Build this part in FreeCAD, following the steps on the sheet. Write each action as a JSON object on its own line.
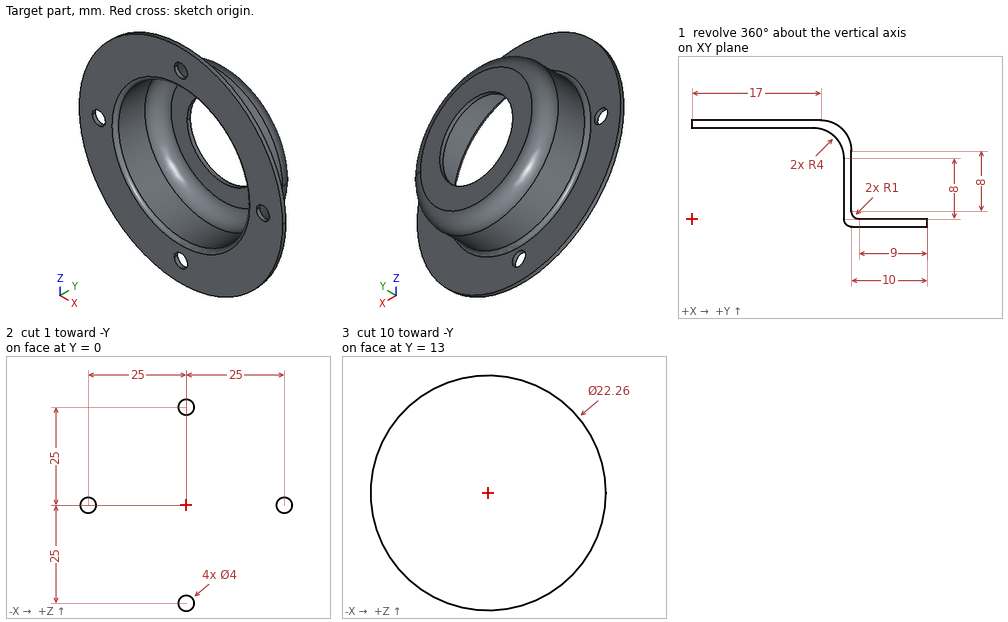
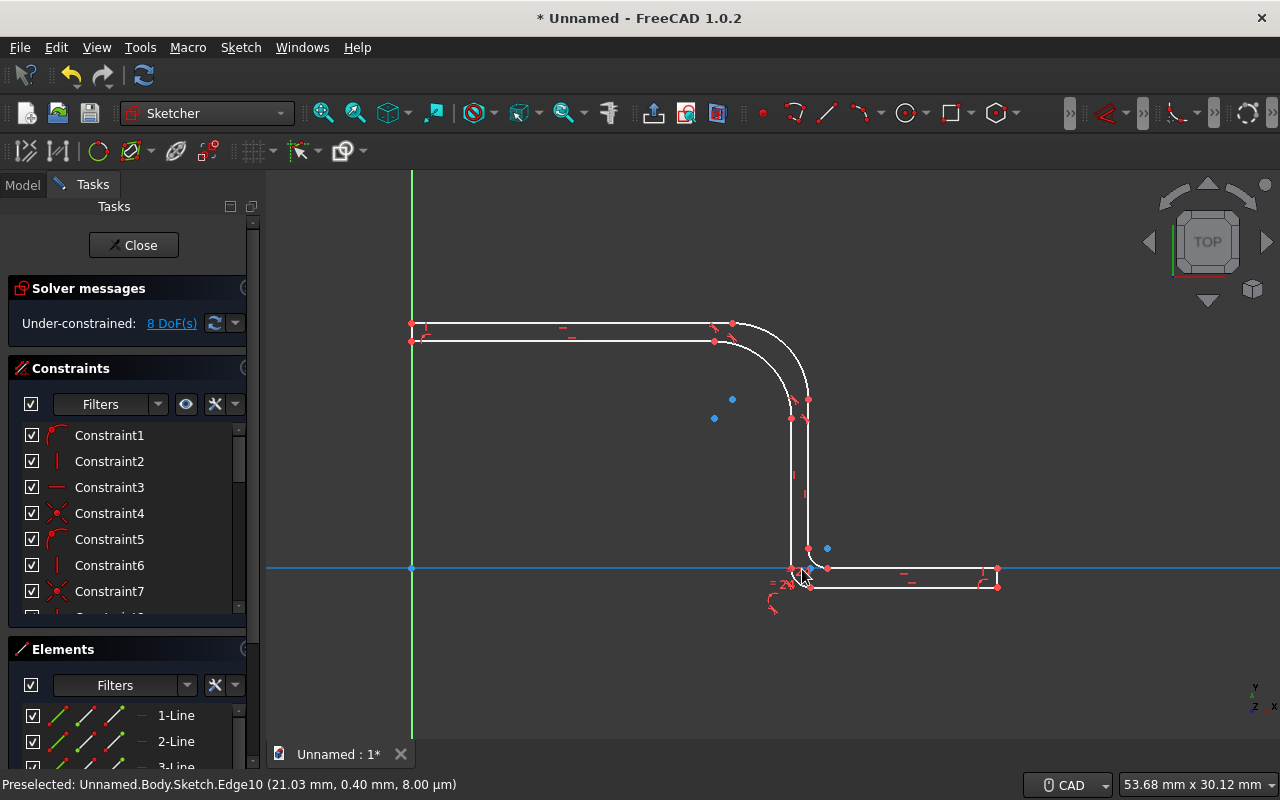
{"action": "left_click", "coordinate": [800, 365]}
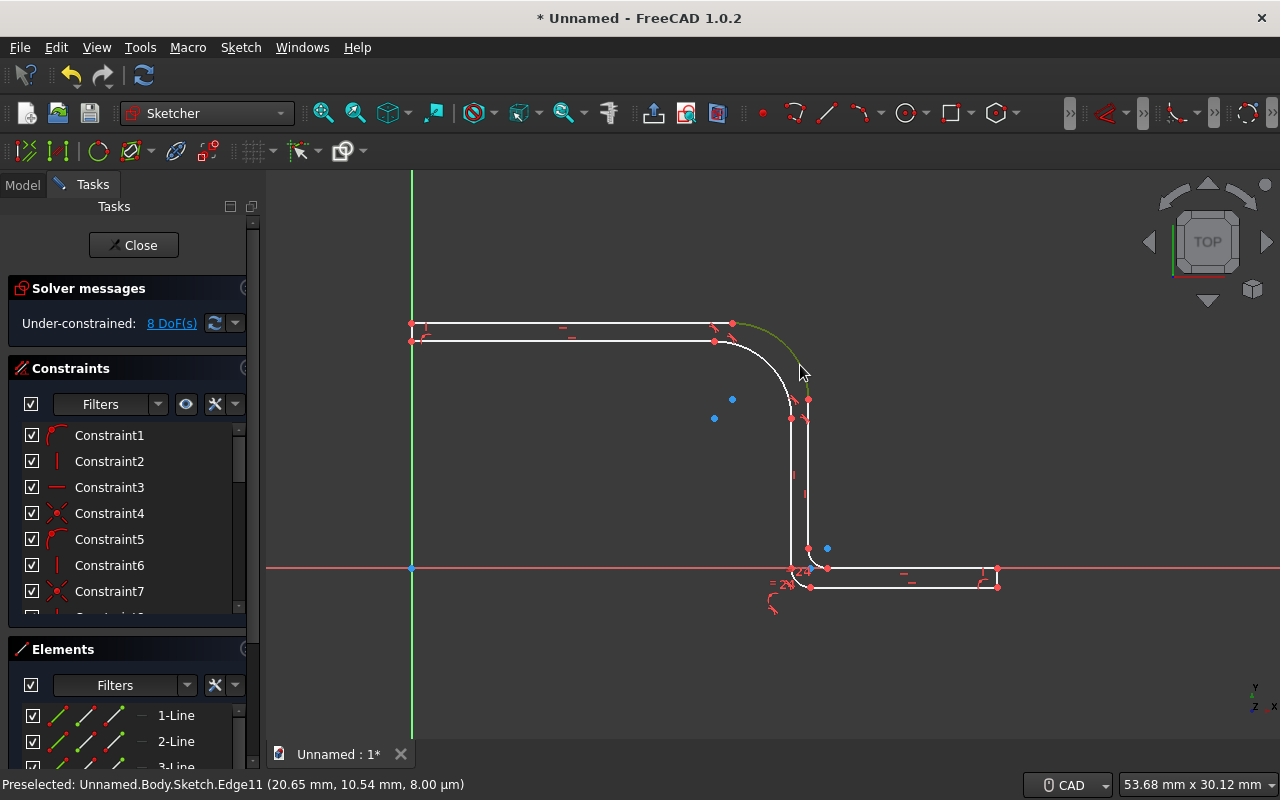
{"action": "left_click", "coordinate": [783, 383]}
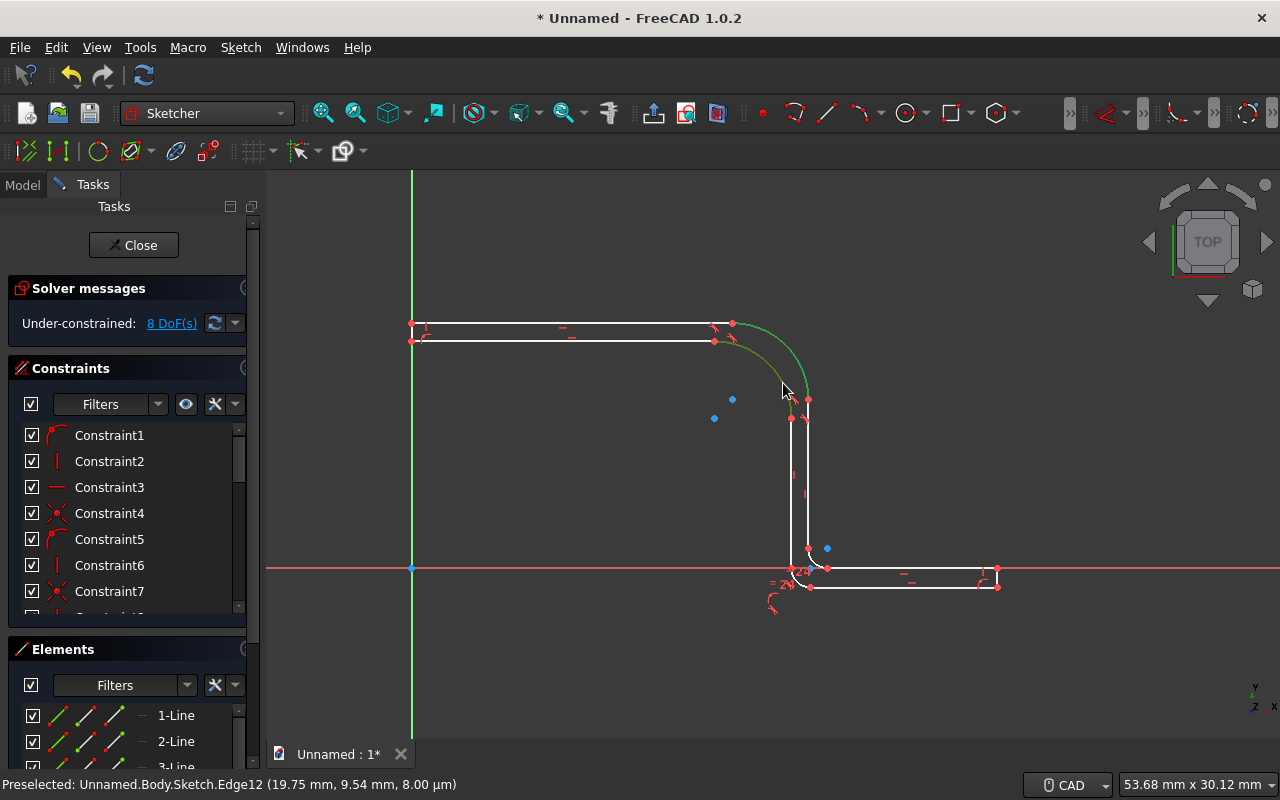
{"action": "key", "text": "e"}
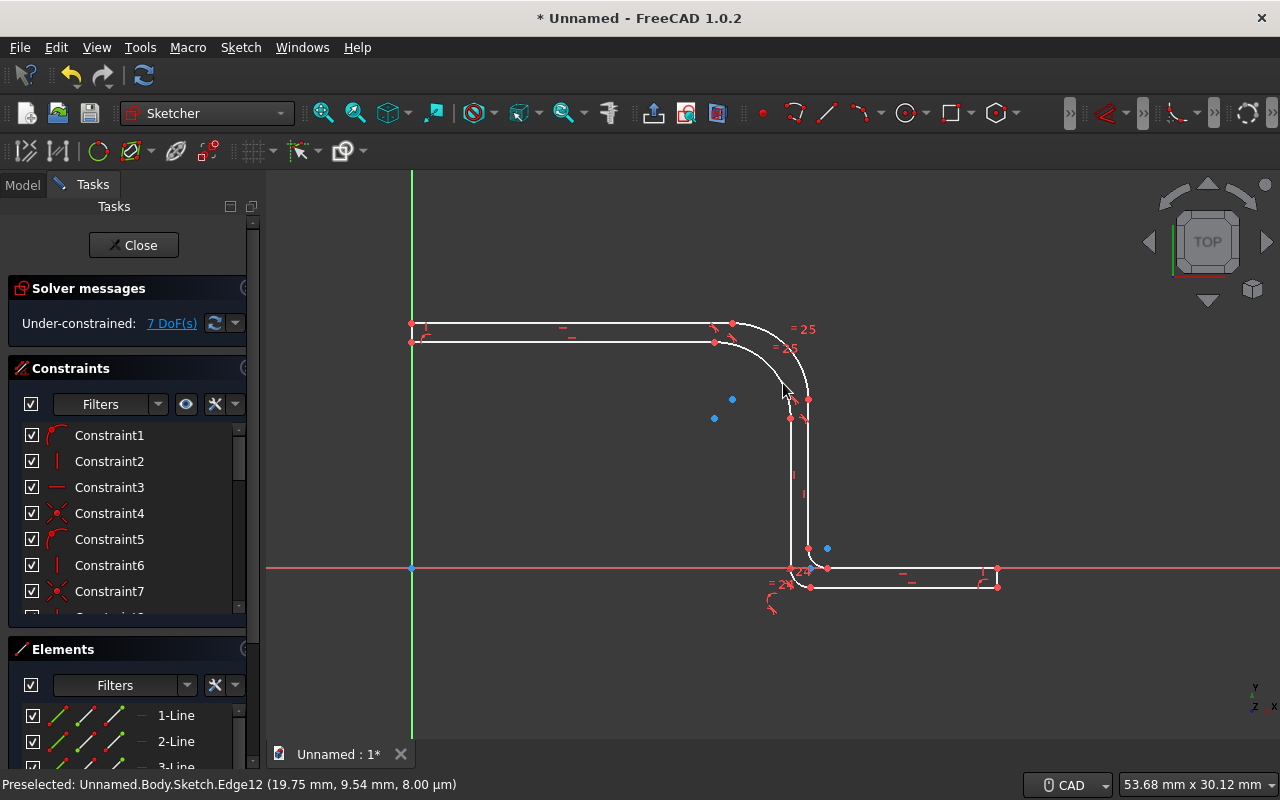
{"action": "left_click", "coordinate": [1106, 114]}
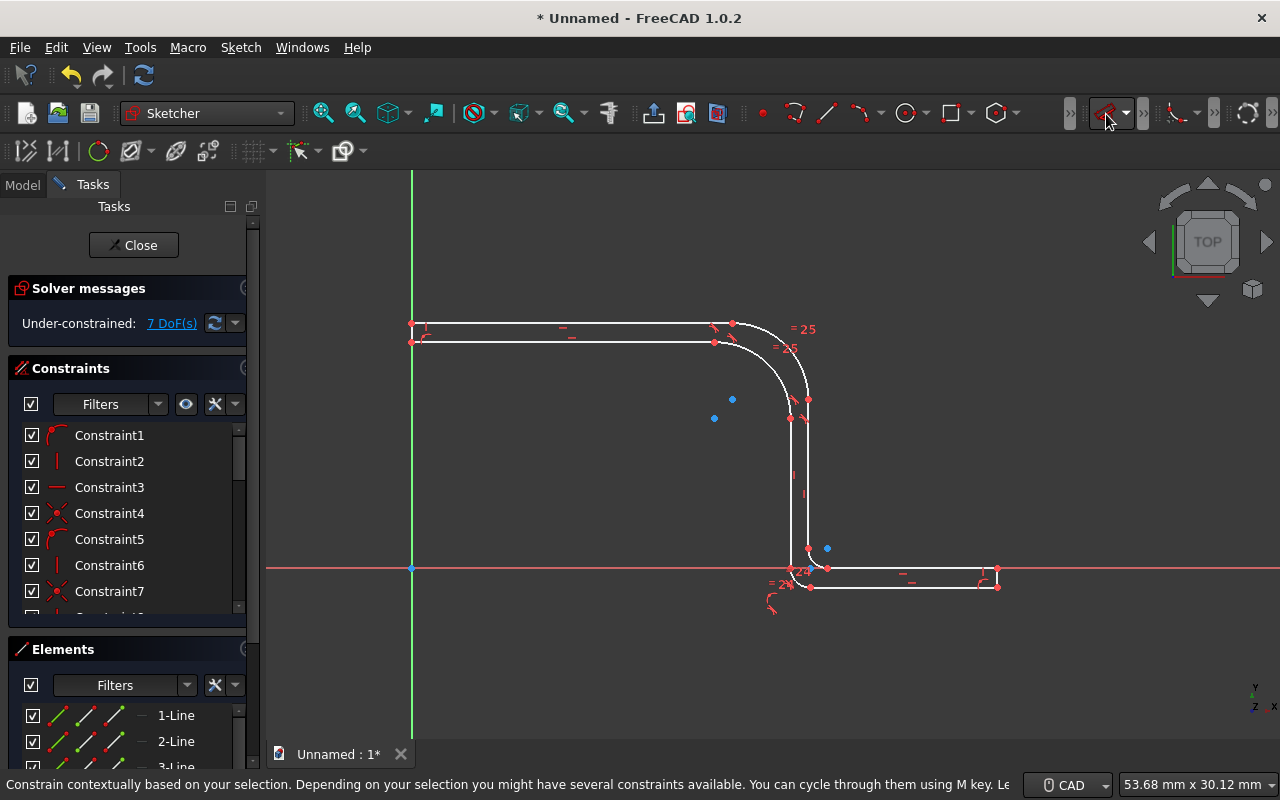
{"action": "scroll", "coordinate": [801, 585], "scroll_direction": "up", "scroll_amount": 4}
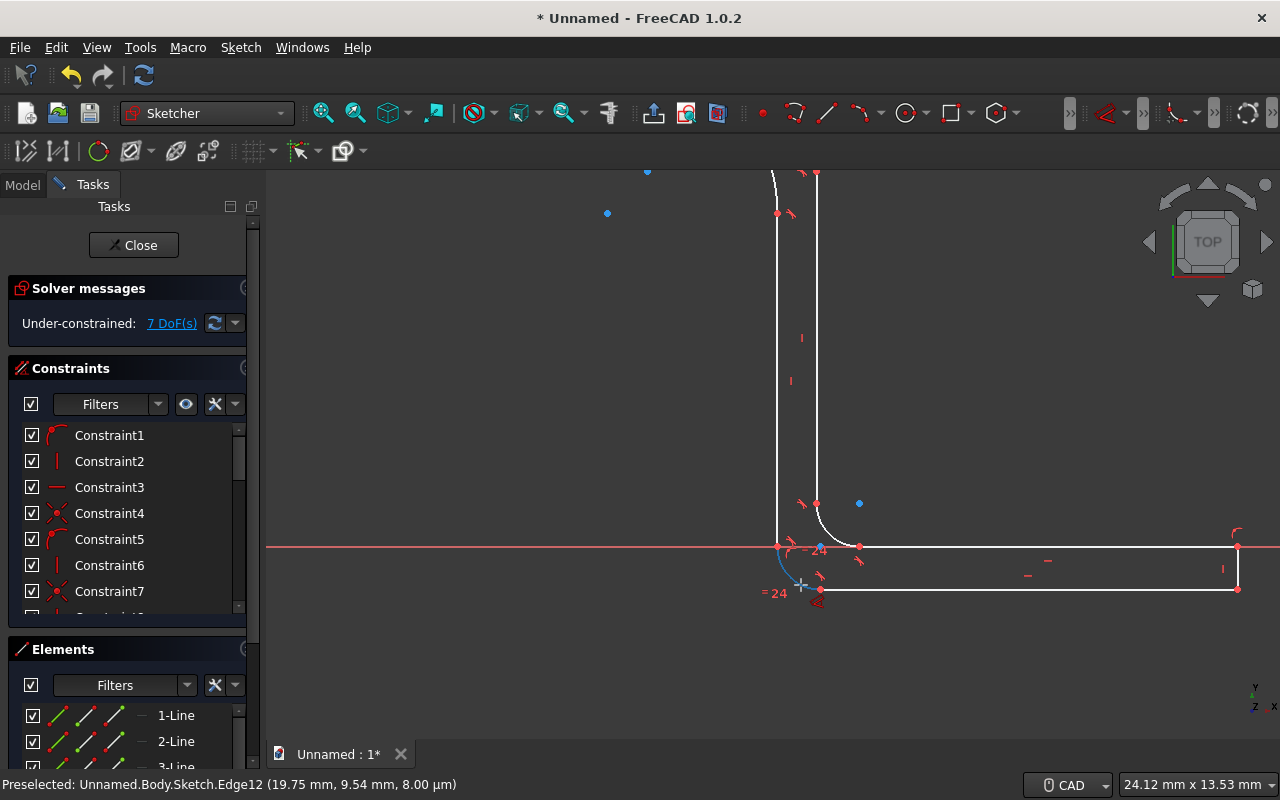
{"action": "left_click", "coordinate": [801, 585]}
{"action": "left_click", "coordinate": [787, 614]}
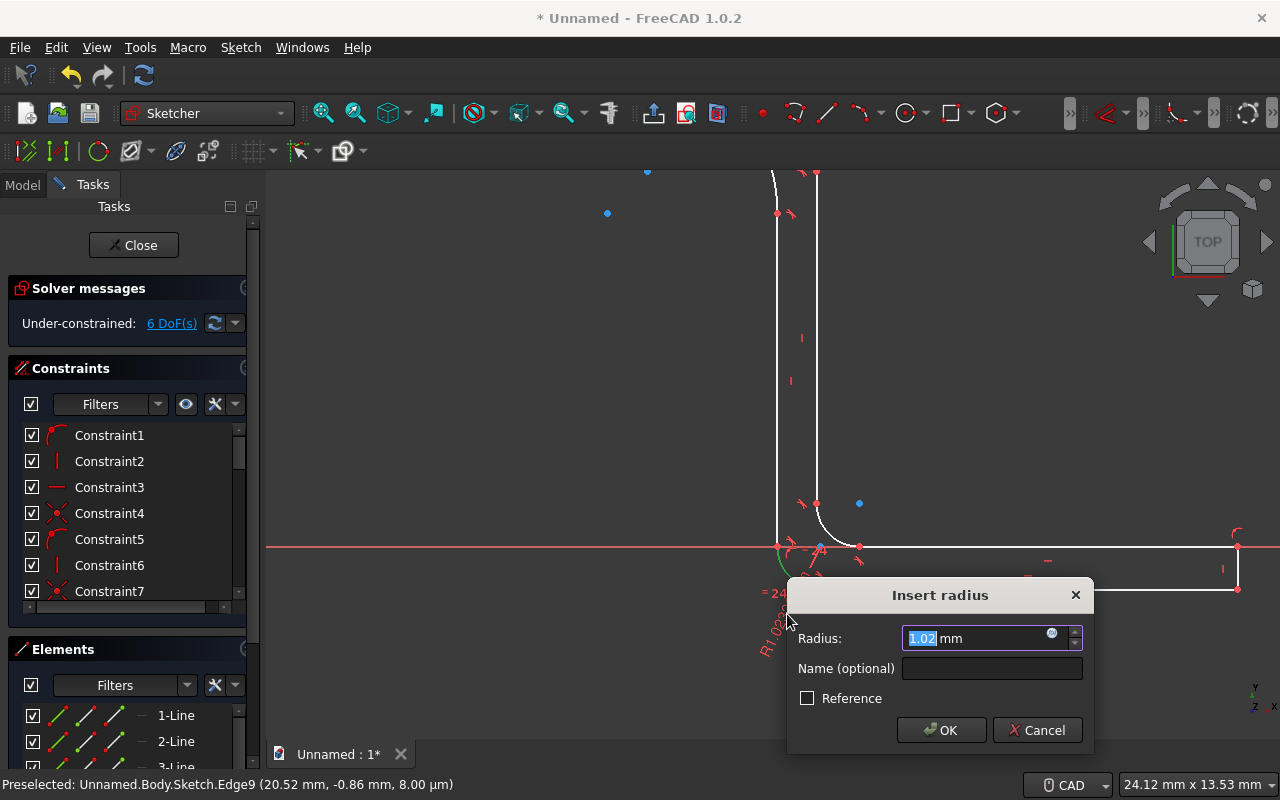
{"action": "type", "text": "1"}
{"action": "key", "text": "Return"}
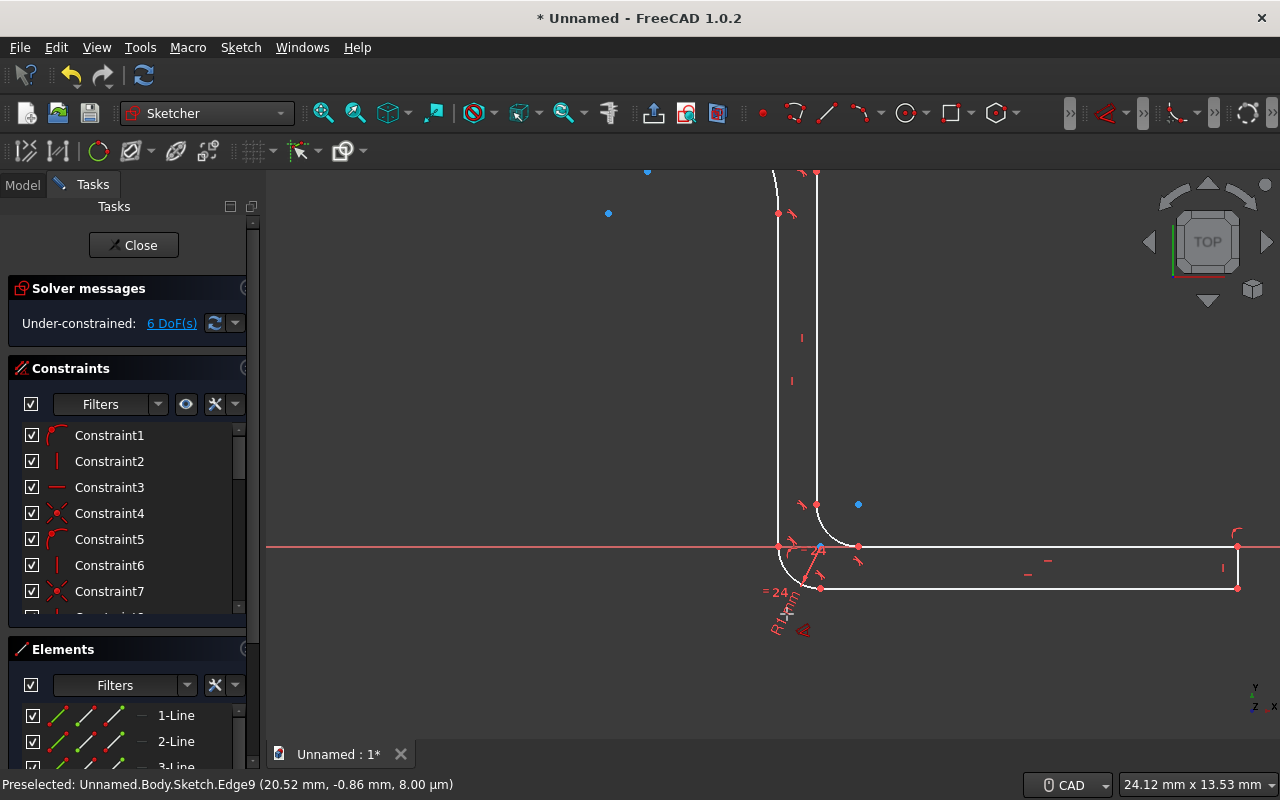
{"action": "scroll", "coordinate": [801, 585], "scroll_direction": "down", "scroll_amount": 4}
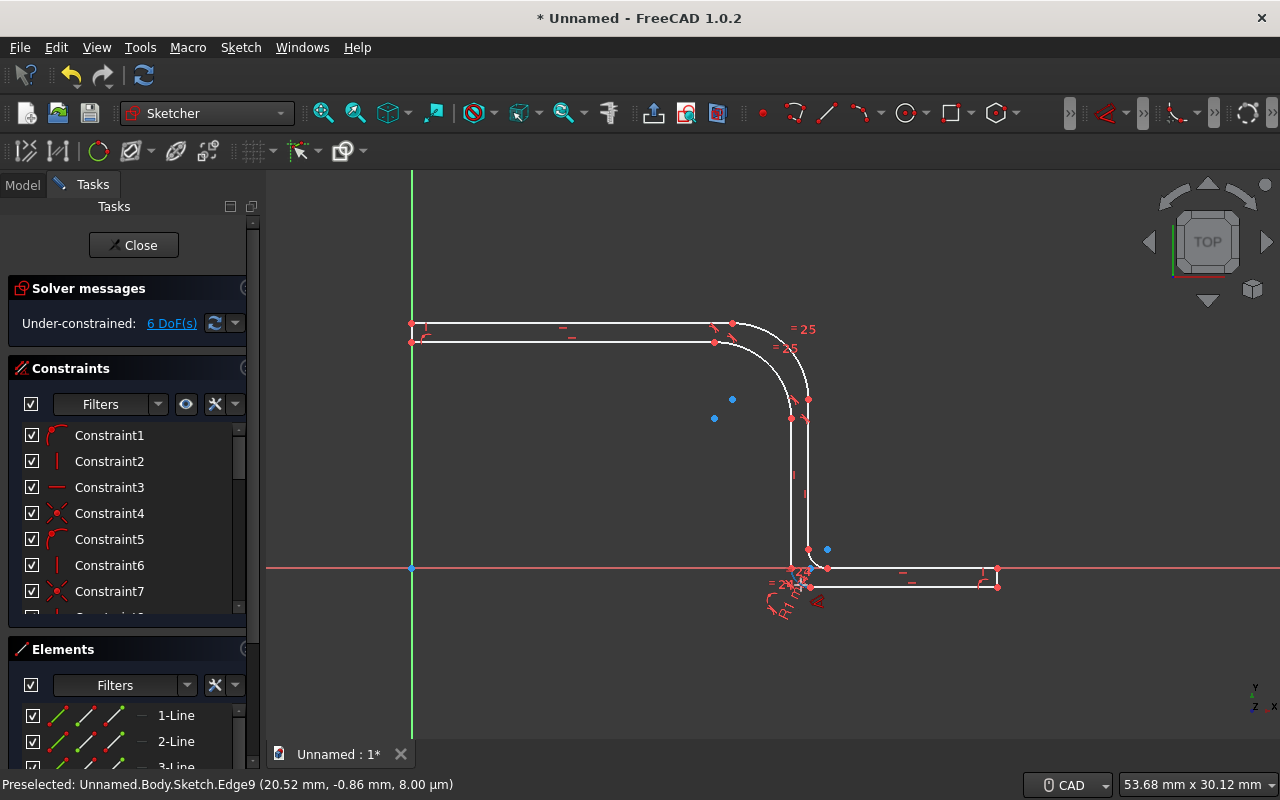
{"action": "left_click", "coordinate": [800, 365]}
{"action": "left_click", "coordinate": [829, 351]}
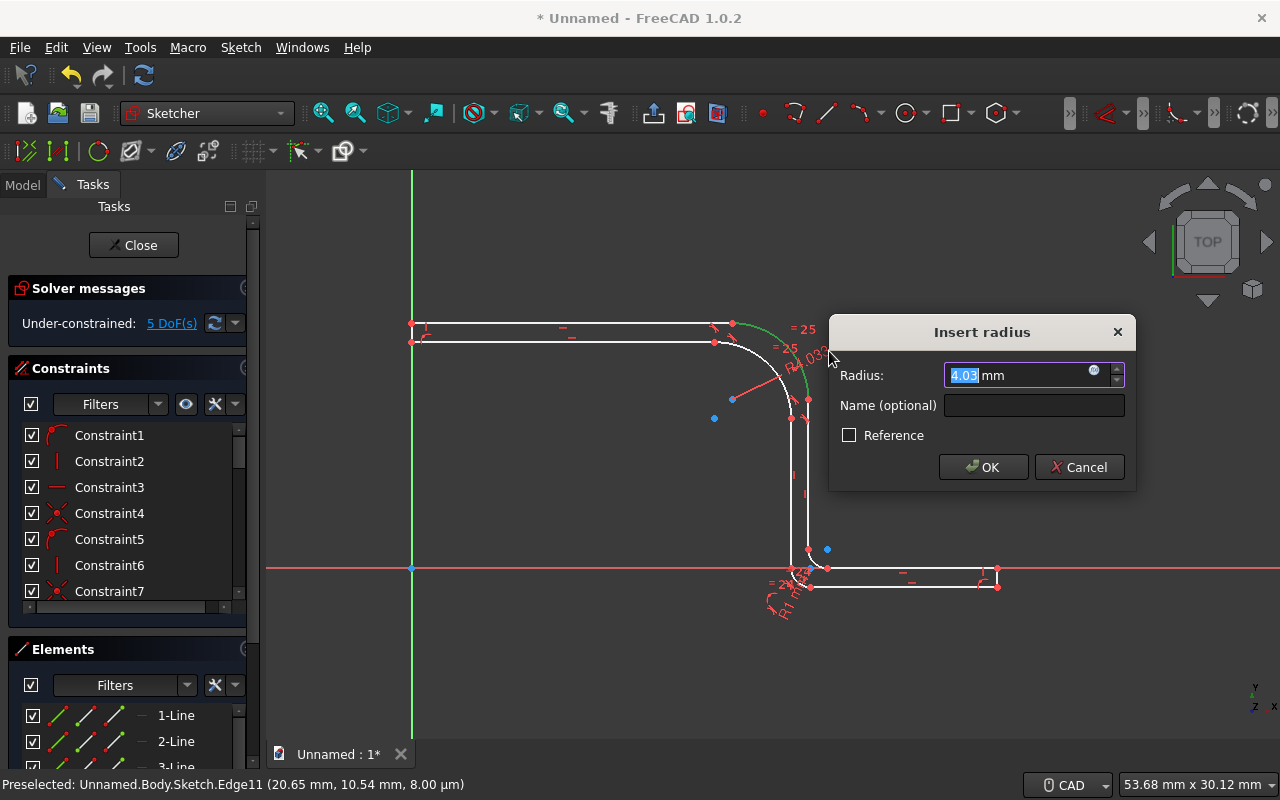
{"action": "type", "text": "4"}
{"action": "key", "text": "Return"}